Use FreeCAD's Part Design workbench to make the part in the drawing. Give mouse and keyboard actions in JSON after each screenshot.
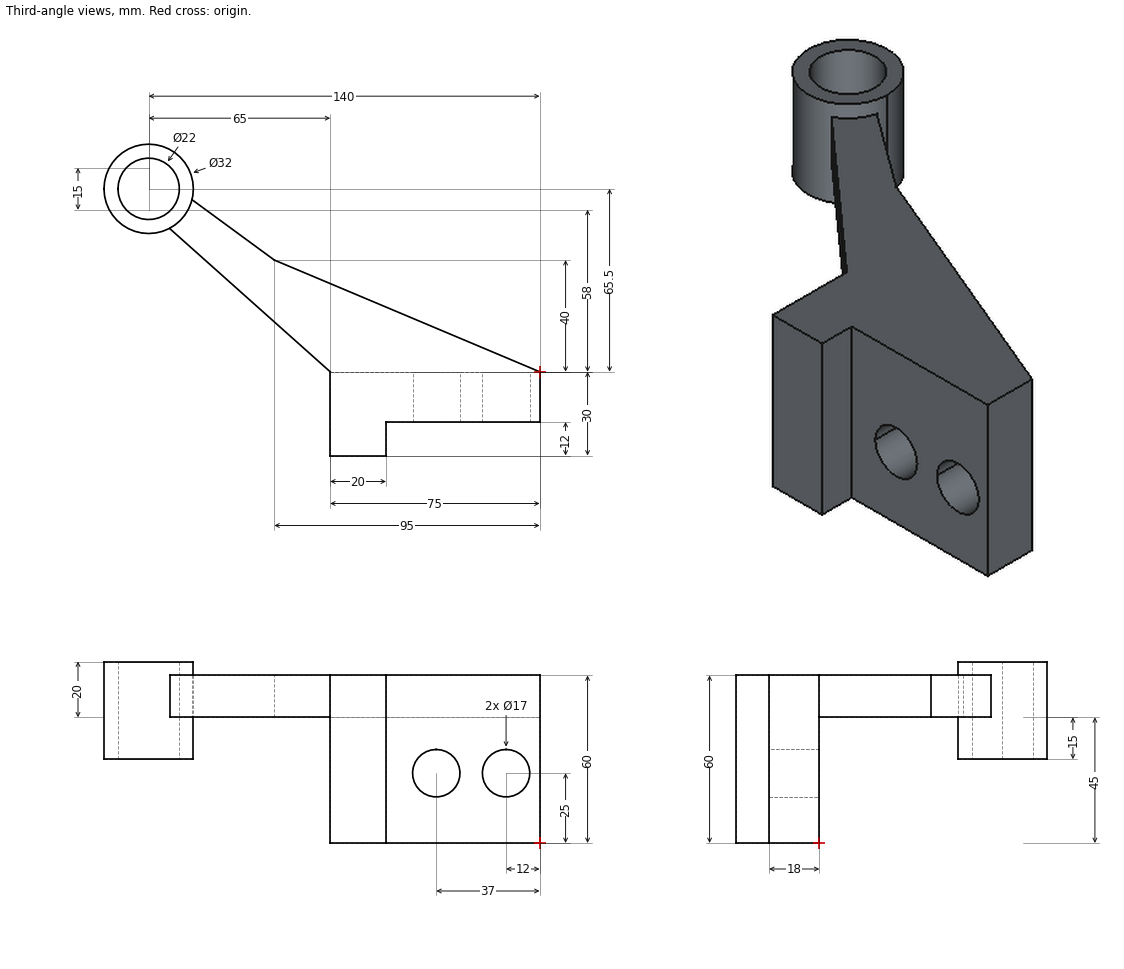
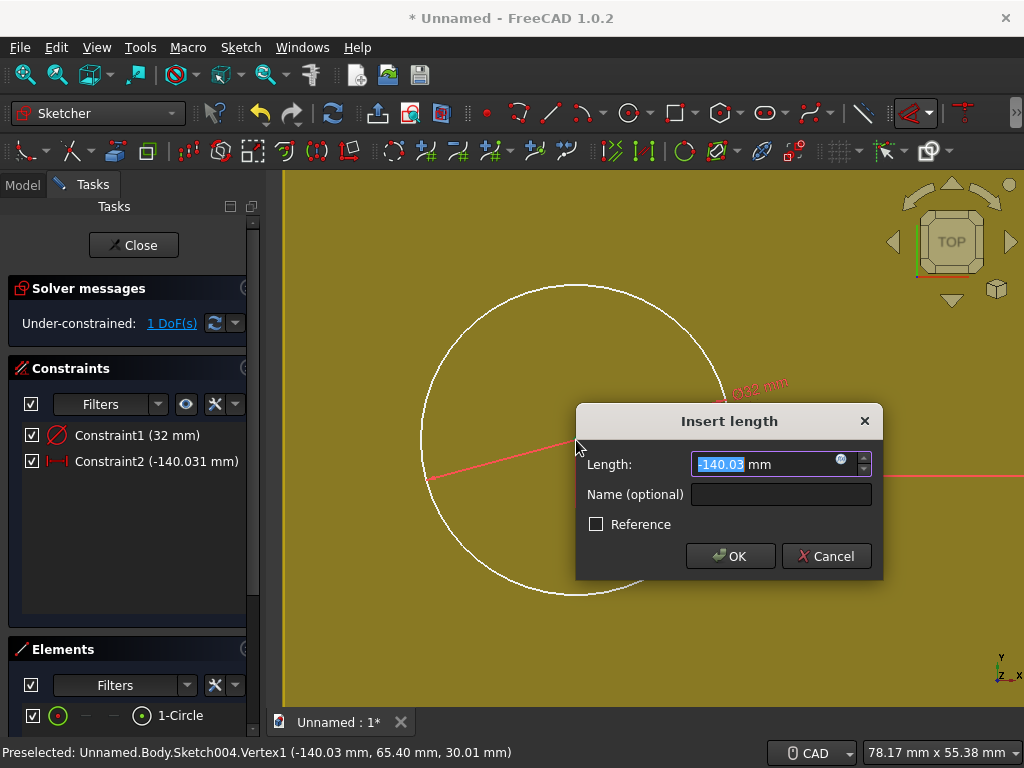
{"action": "type", "text": "-140"}
{"action": "key", "text": "Return"}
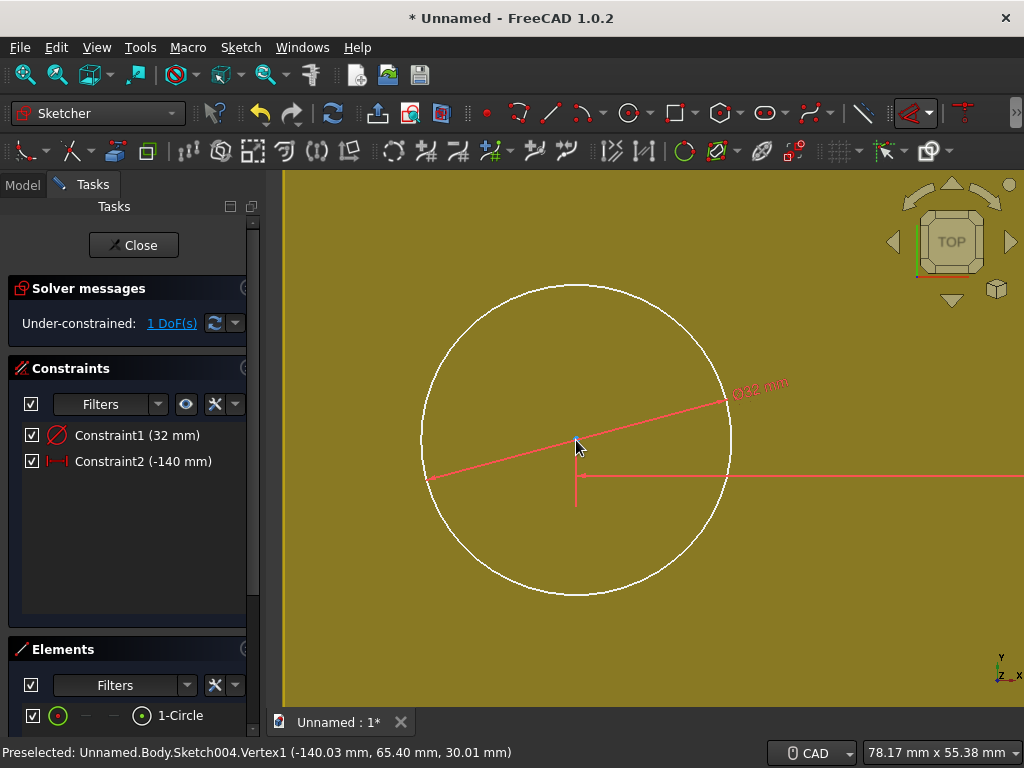
{"action": "left_click", "coordinate": [576, 440]}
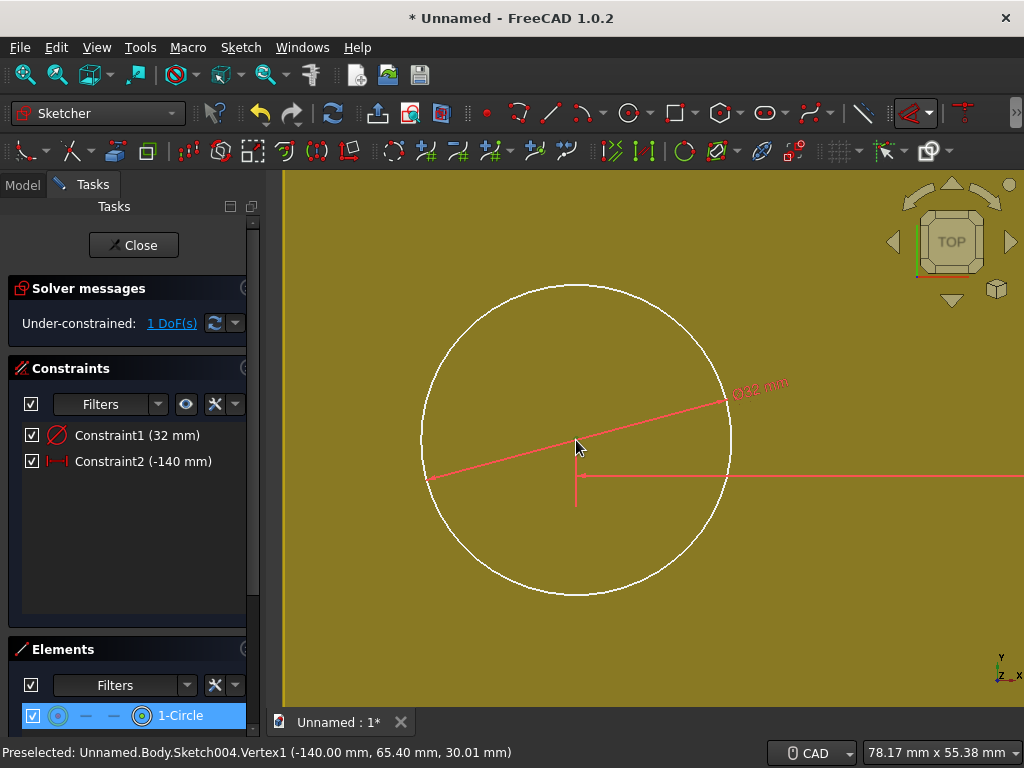
{"action": "left_click", "coordinate": [932, 114]}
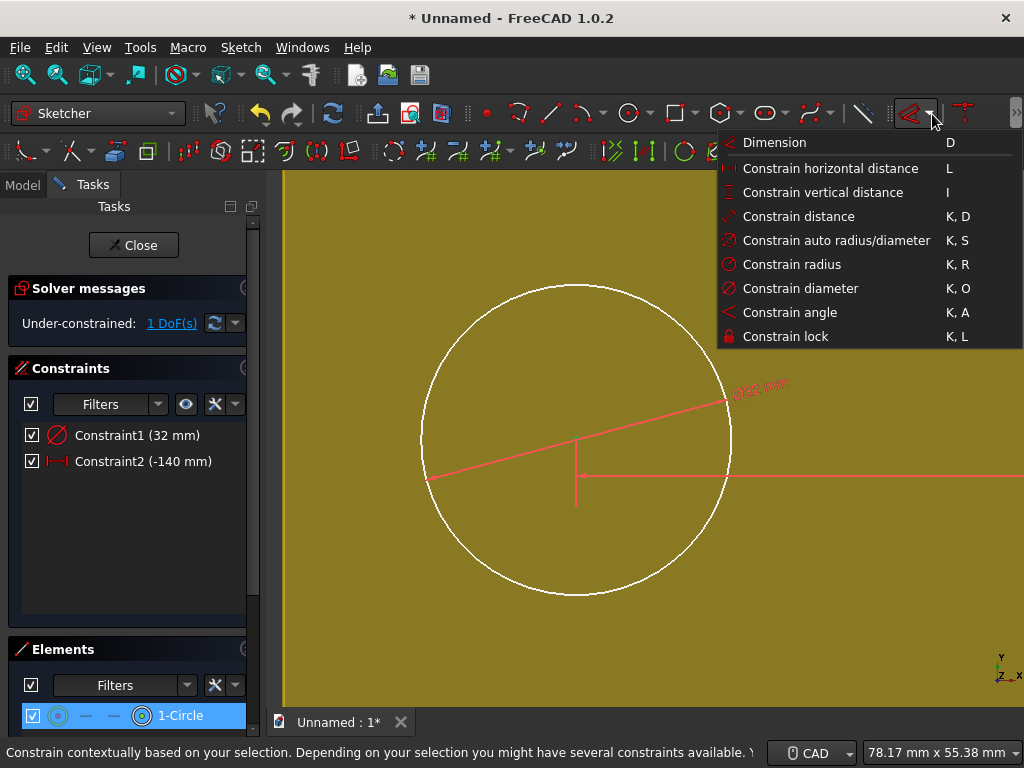
{"action": "left_click", "coordinate": [870, 192]}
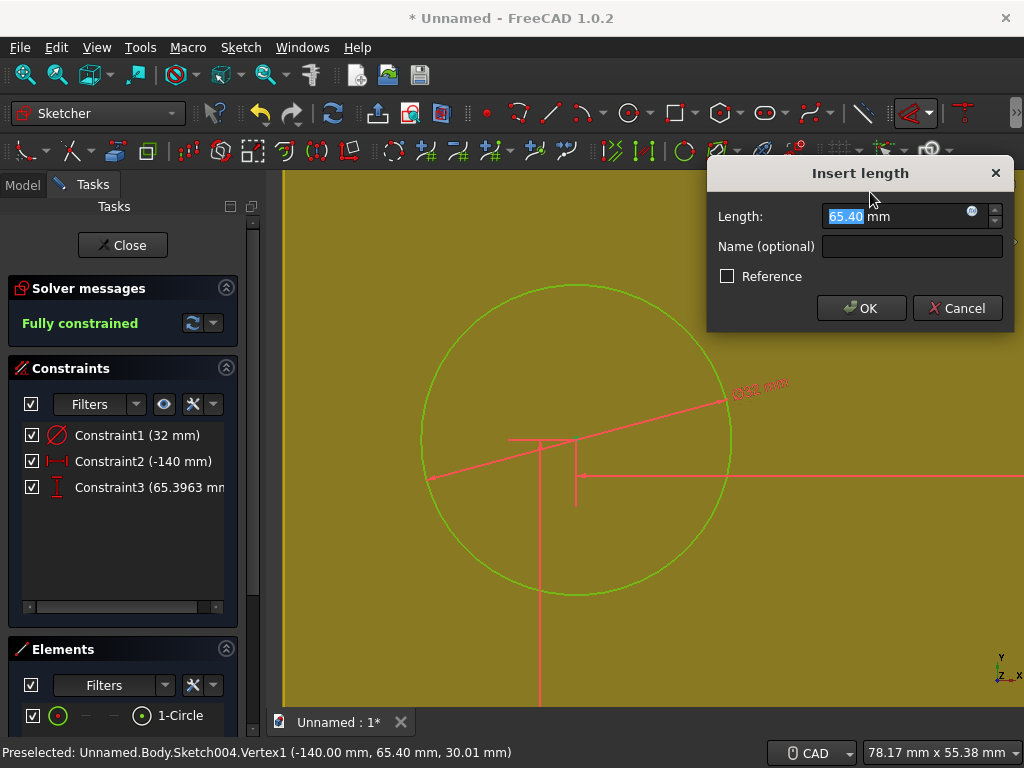
{"action": "type", "text": "65.5"}
{"action": "key", "text": "Return"}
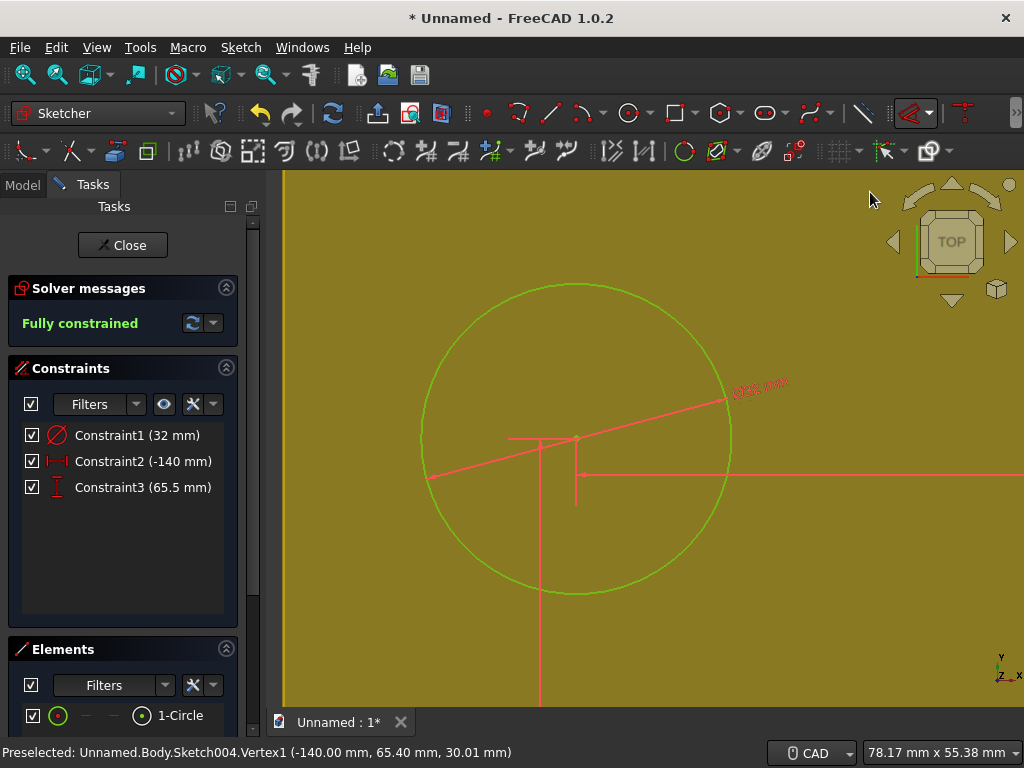
{"action": "left_click", "coordinate": [123, 245]}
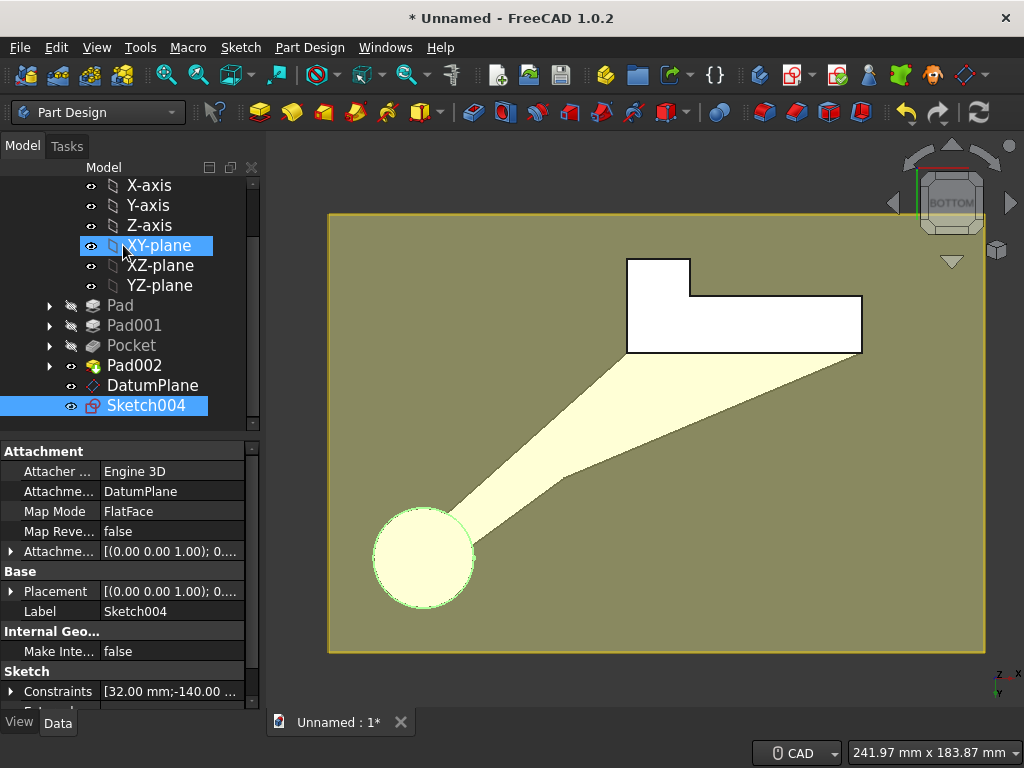
{"action": "left_click", "coordinate": [260, 112]}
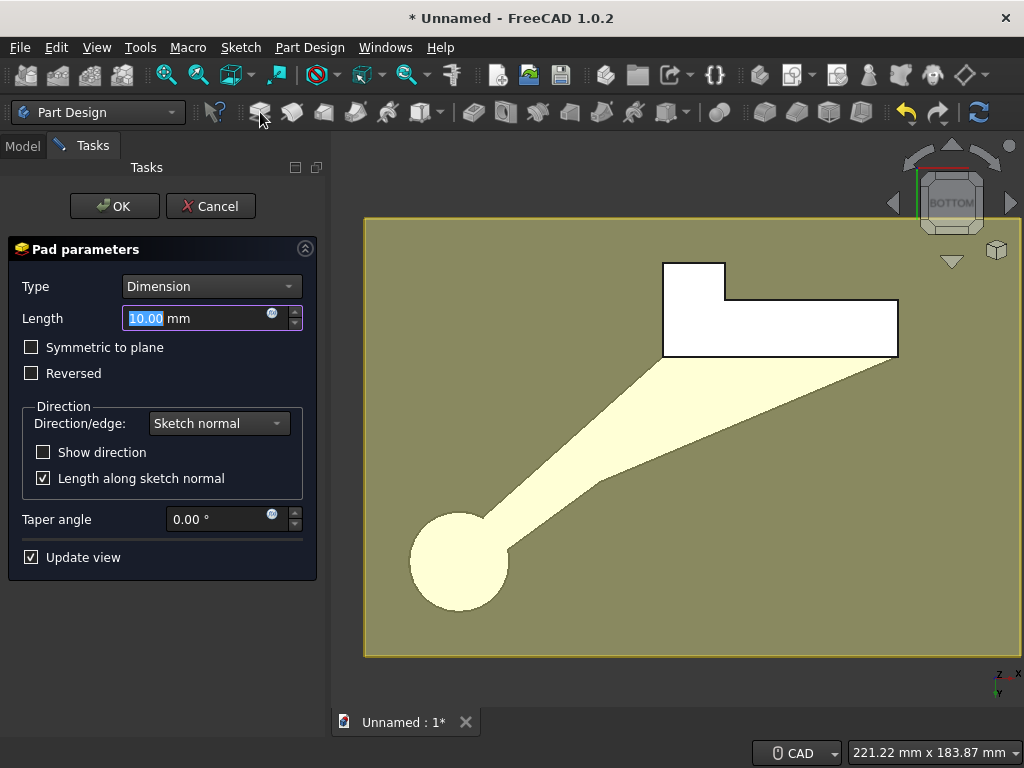
{"action": "type", "text": "15"}
{"action": "key", "text": "Tab"}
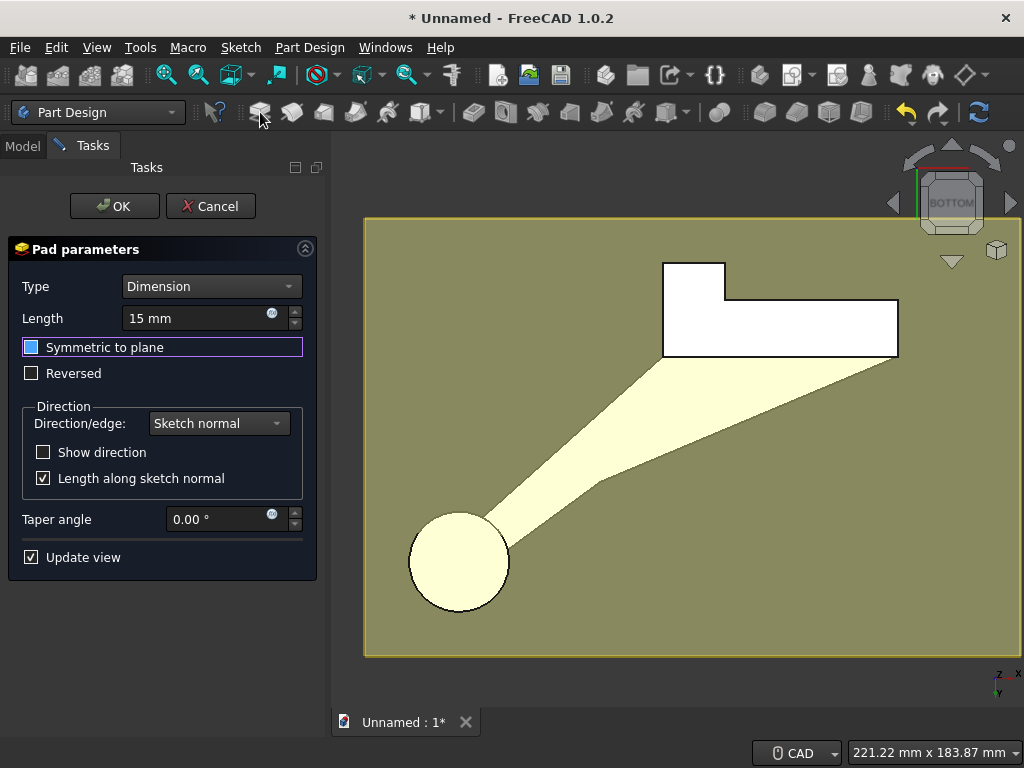
{"action": "left_click", "coordinate": [115, 206]}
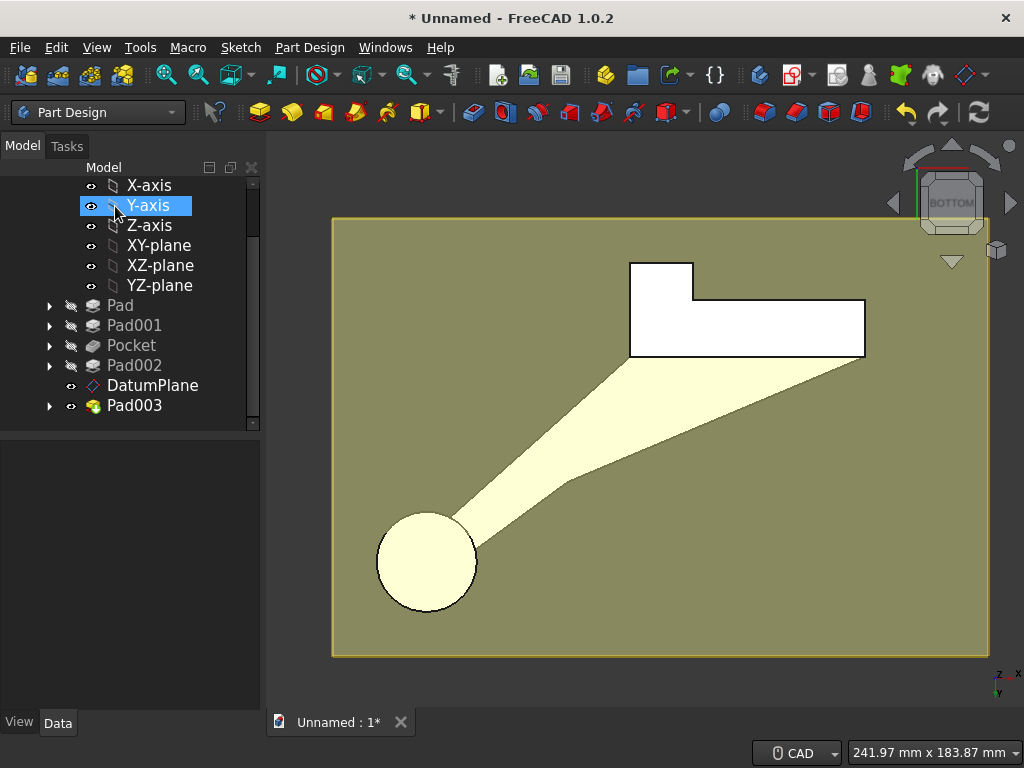
{"action": "left_click", "coordinate": [116, 386]}
{"action": "key", "text": "space"}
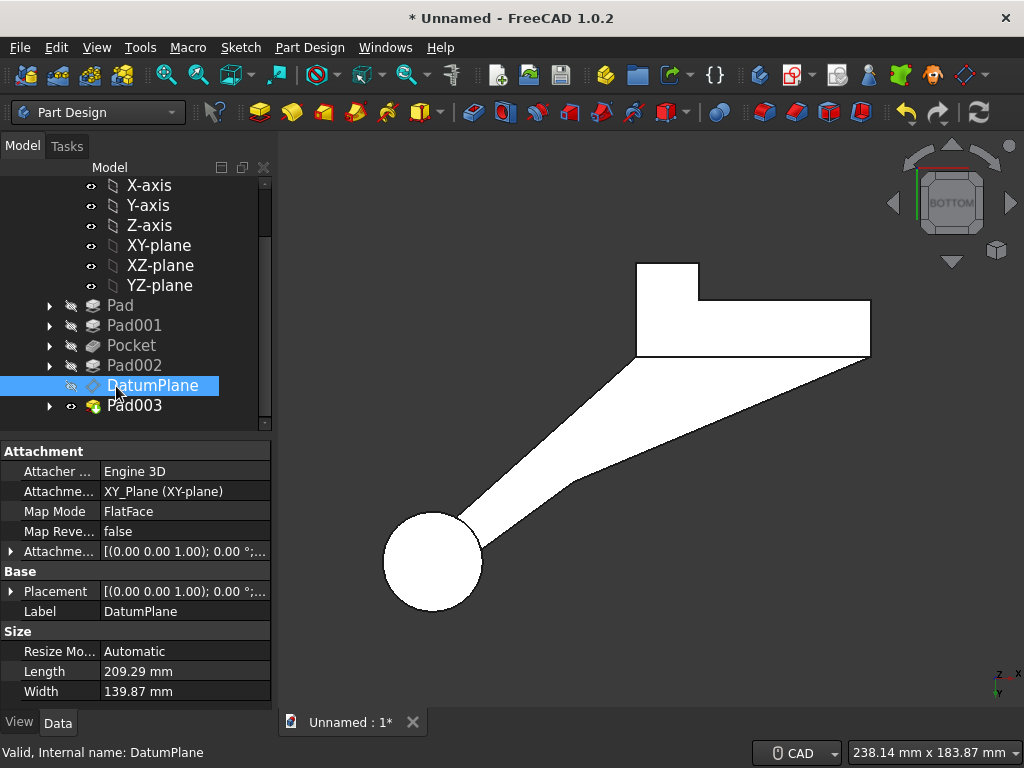
{"action": "left_click", "coordinate": [433, 561]}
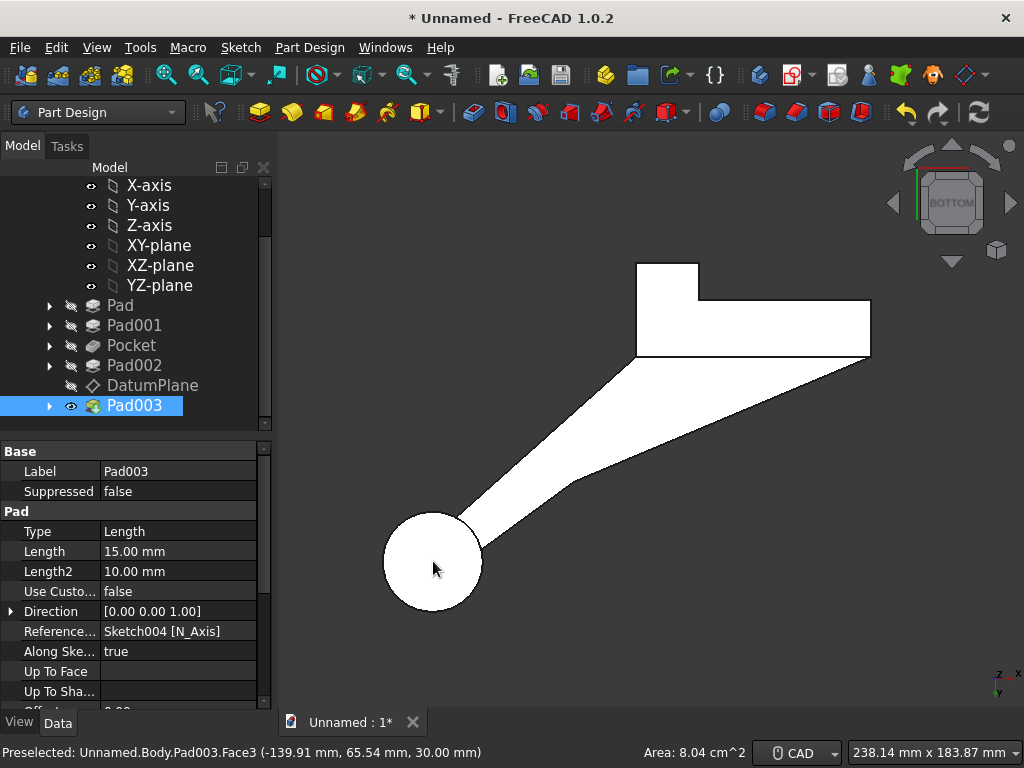
{"action": "left_click", "coordinate": [792, 76]}